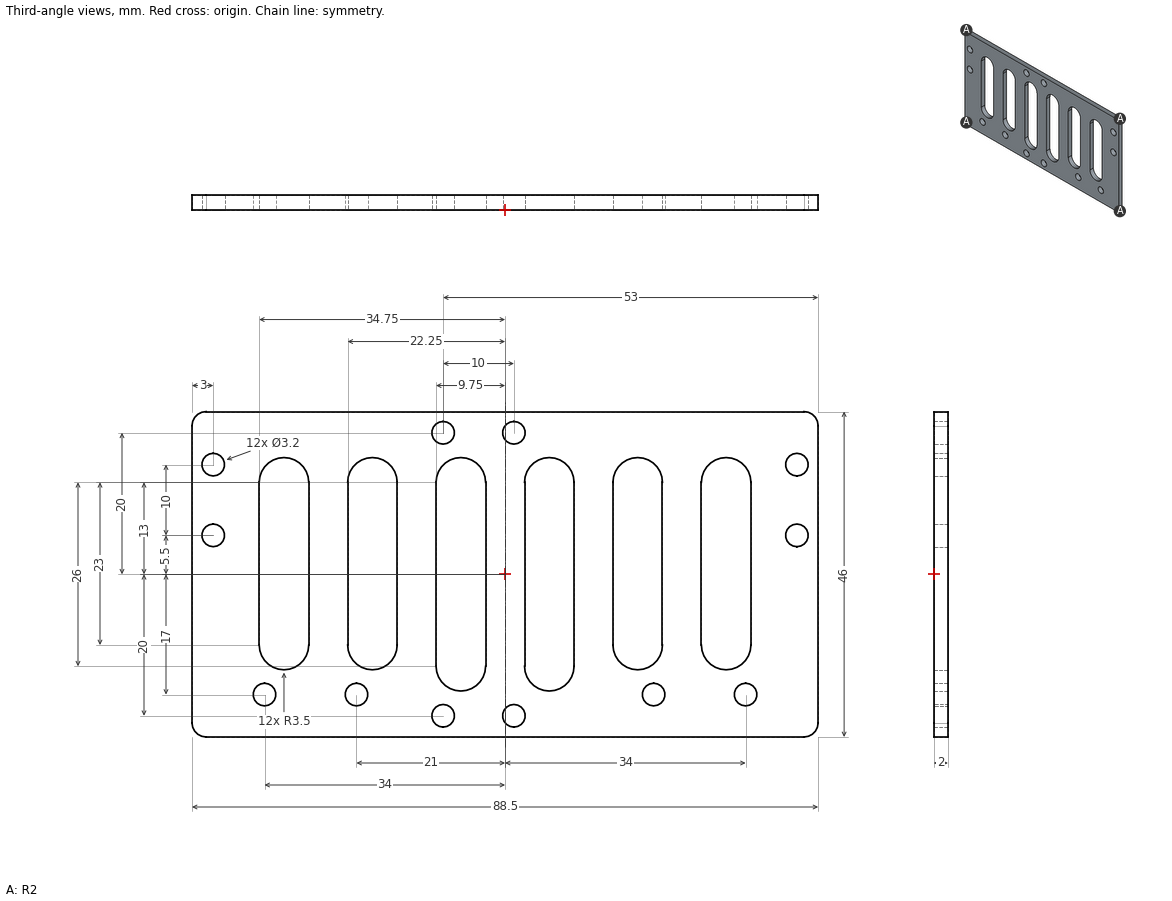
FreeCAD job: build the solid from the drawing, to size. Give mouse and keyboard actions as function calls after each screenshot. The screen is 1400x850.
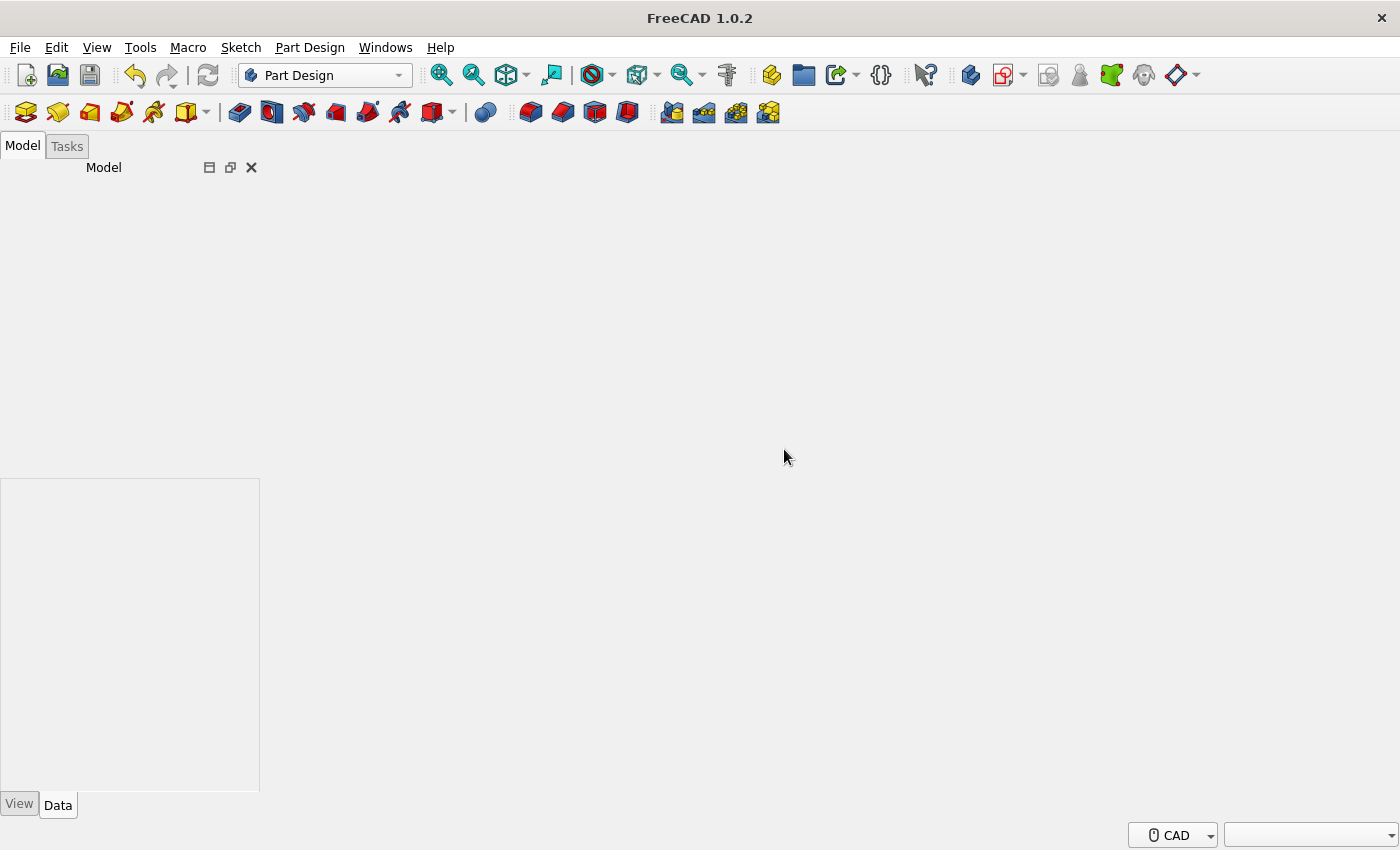
click(26, 76)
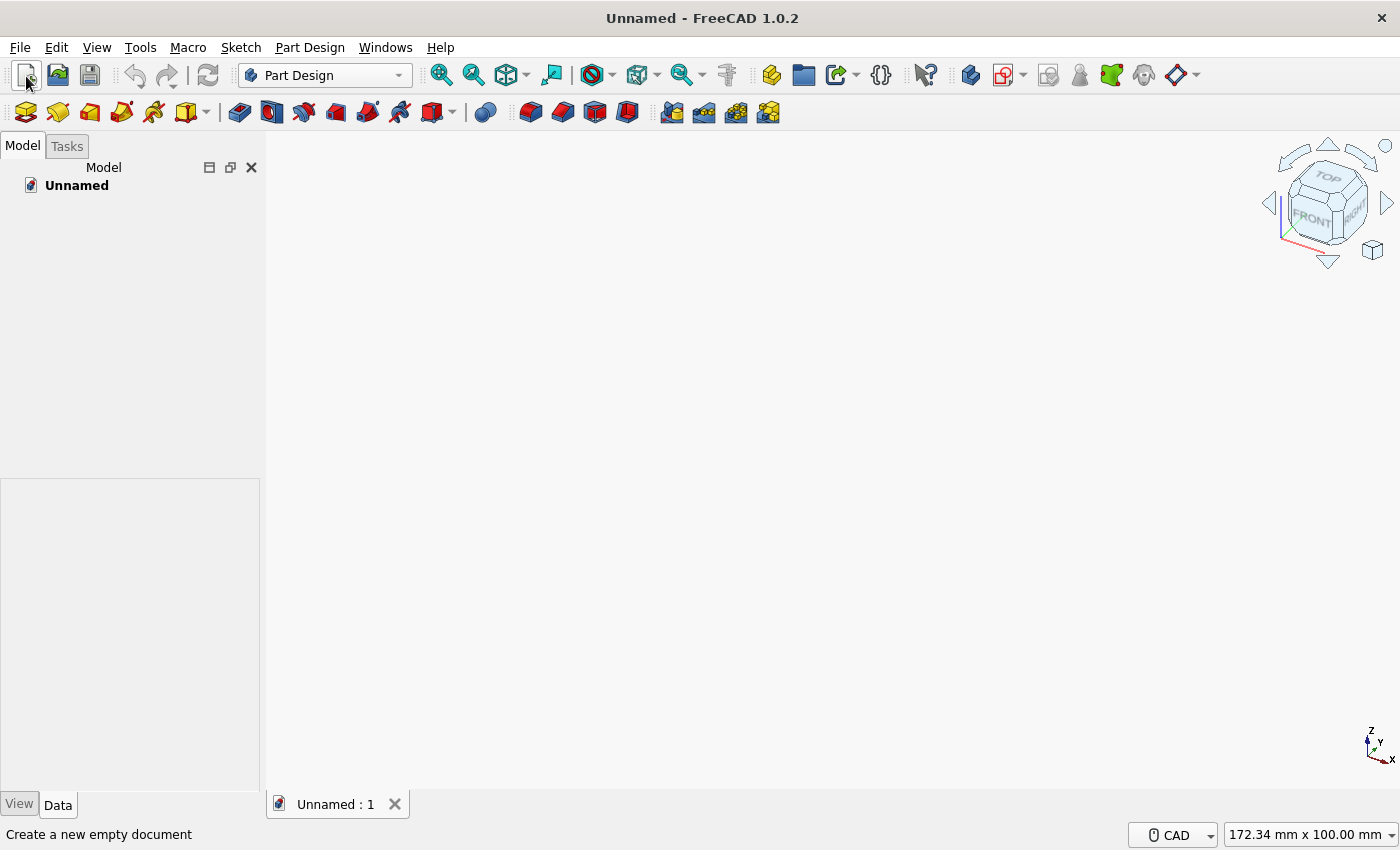
click(1004, 76)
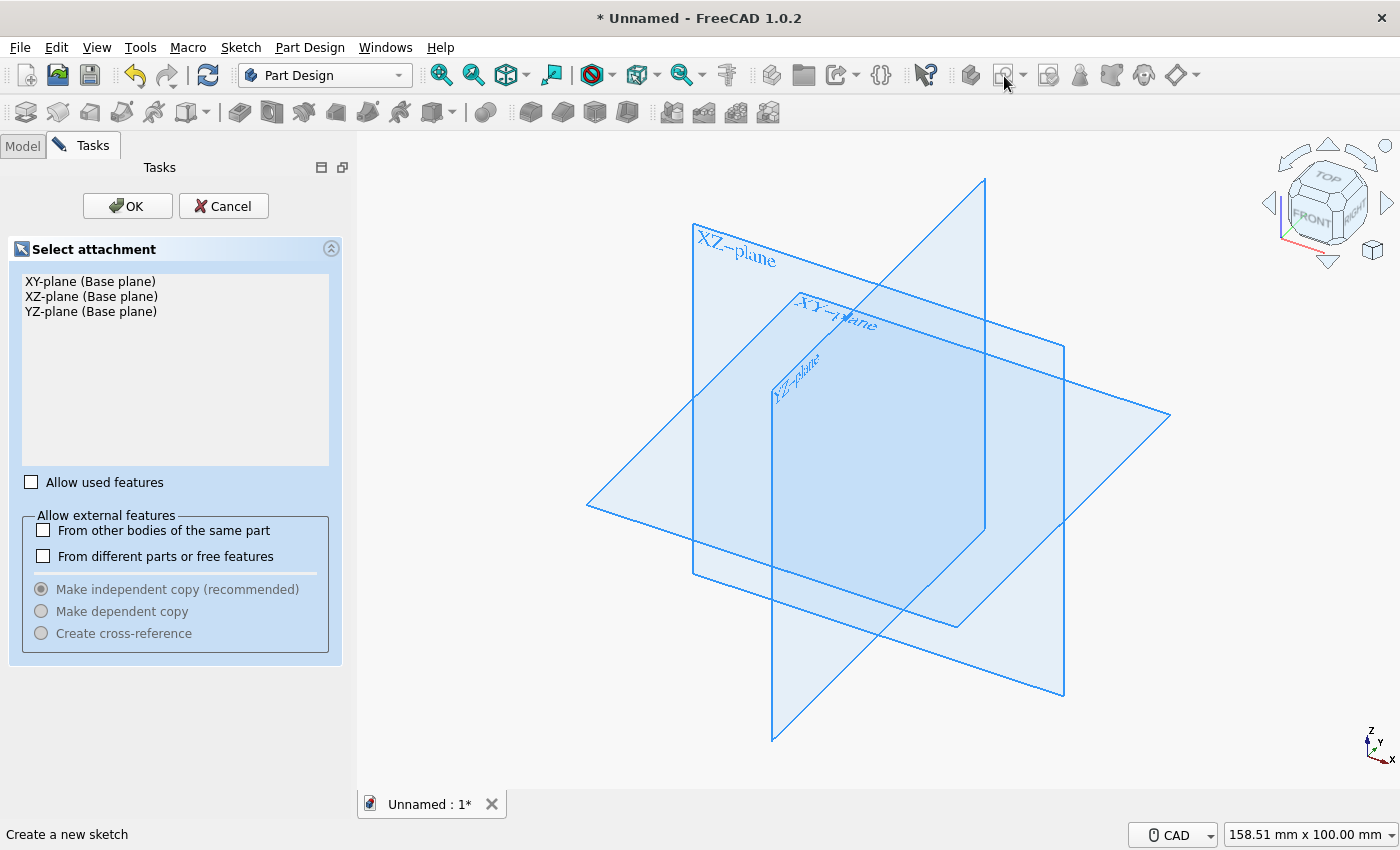
click(82, 296)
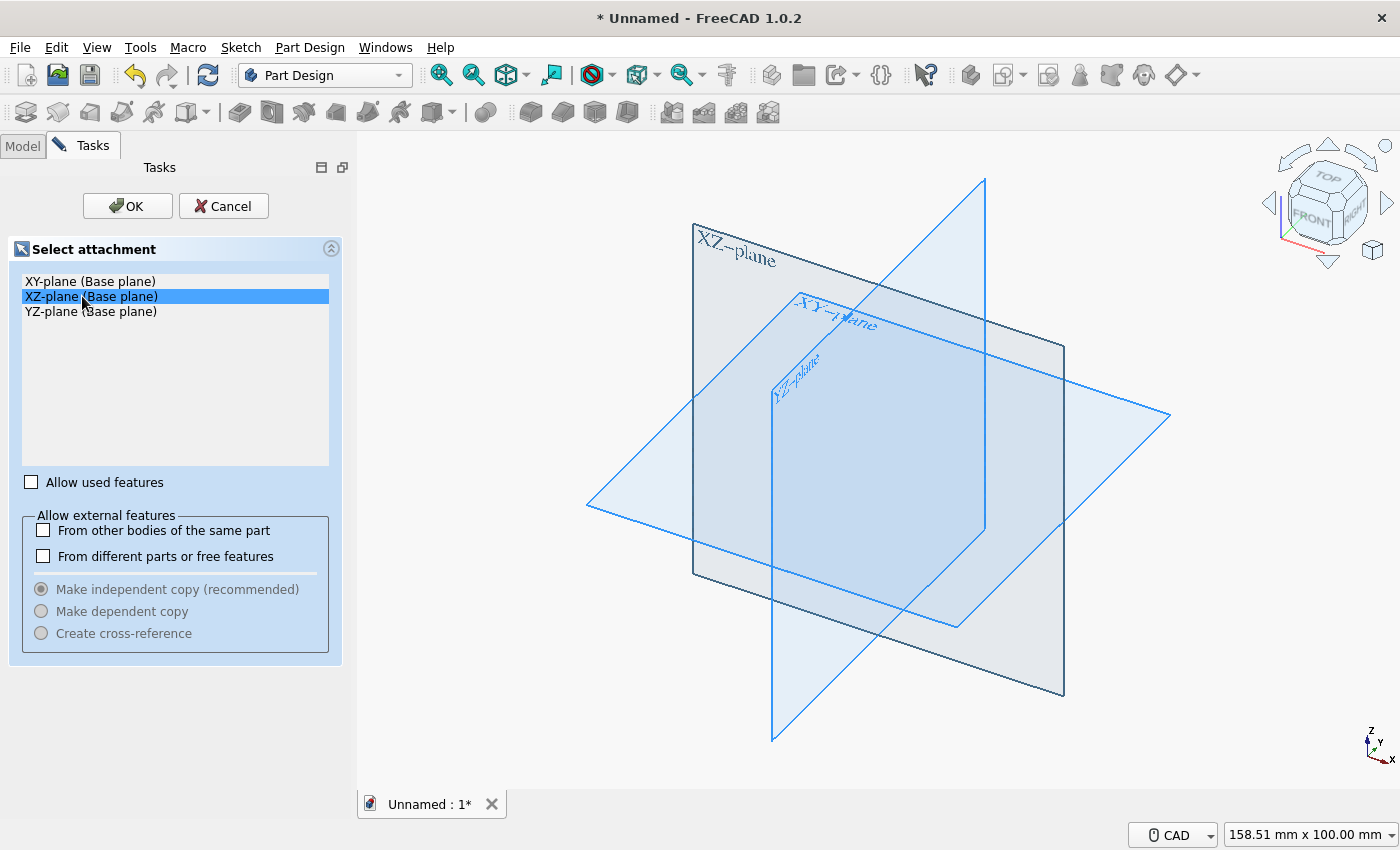
click(128, 206)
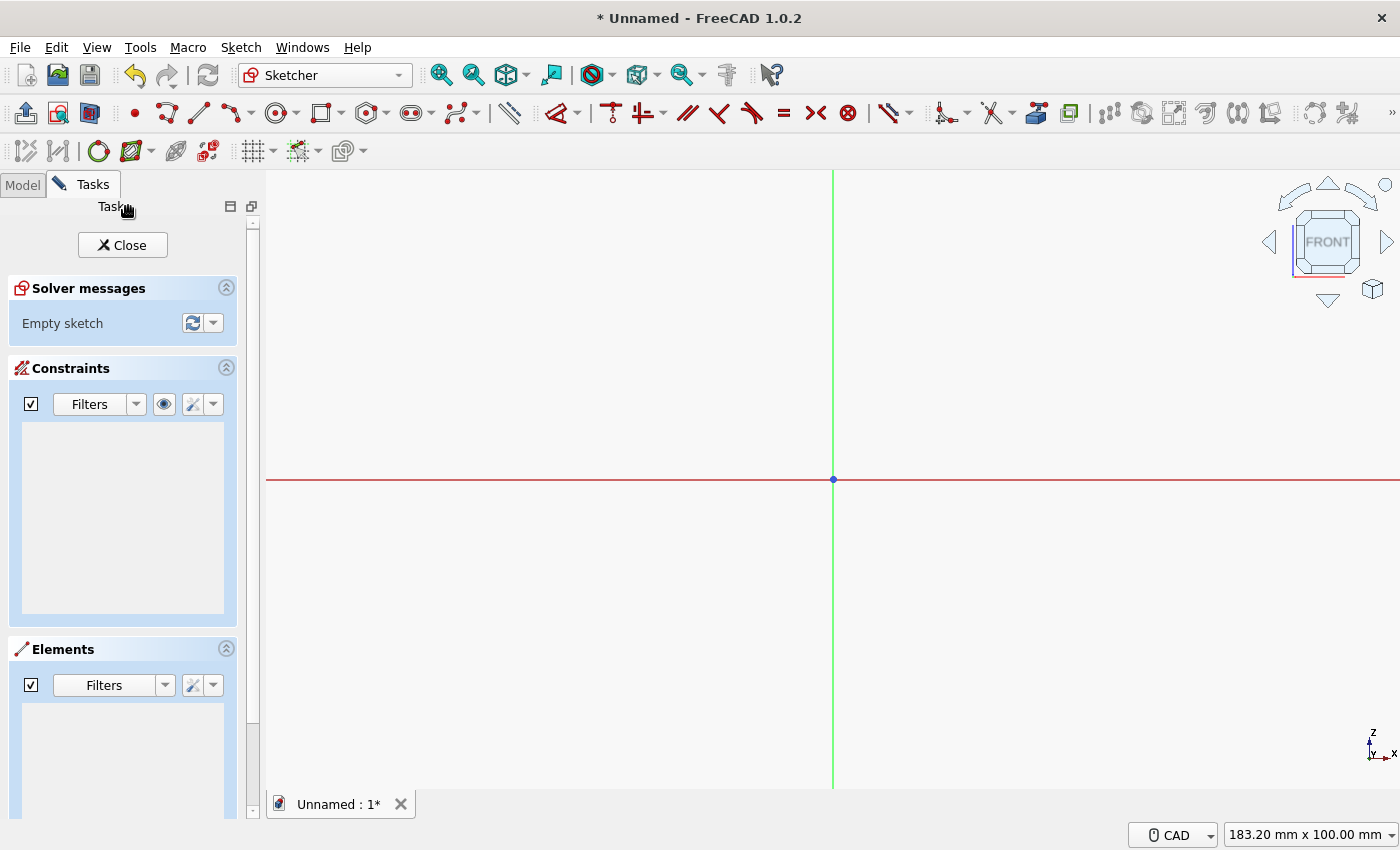
key(g)
key(v)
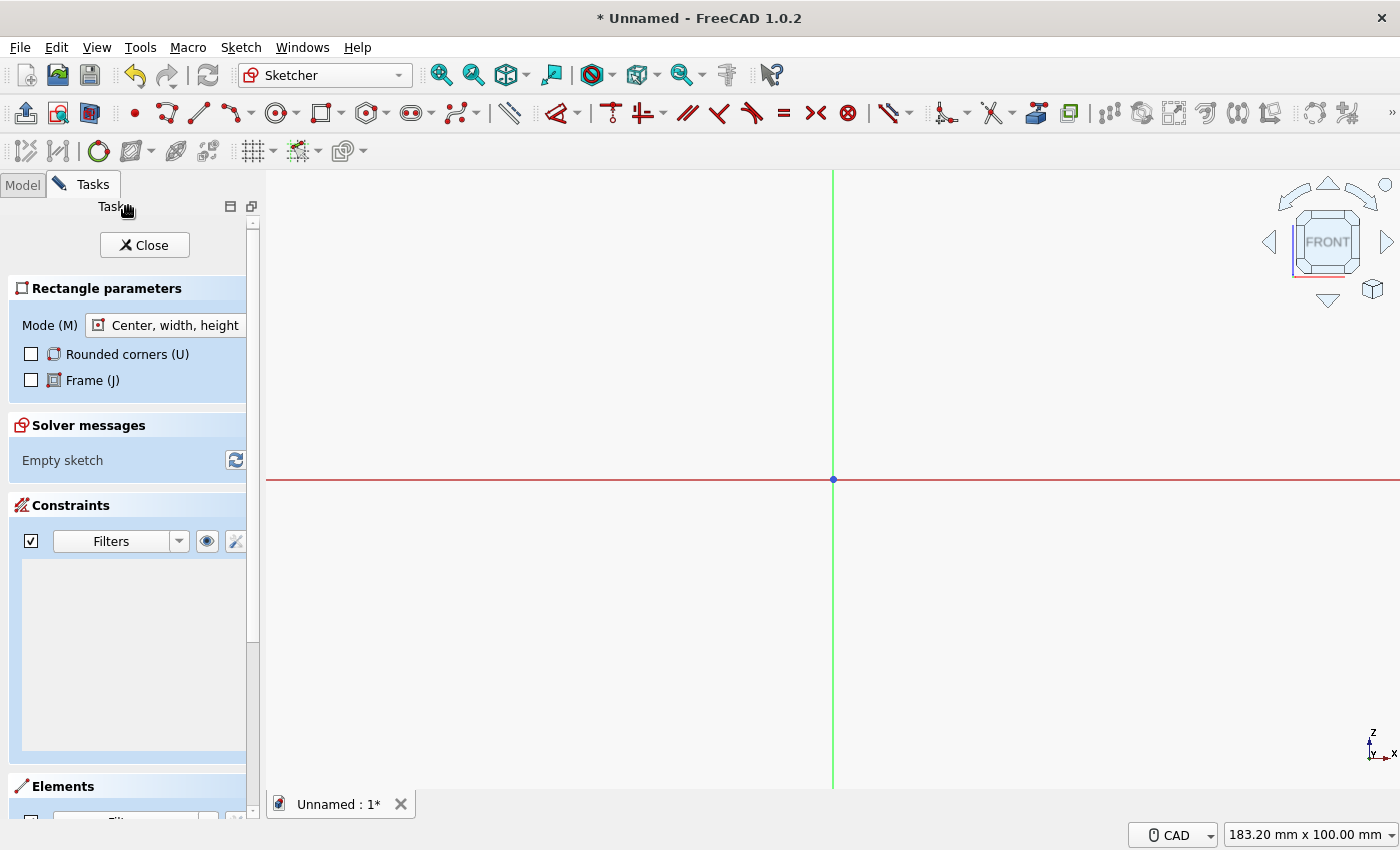
click(833, 480)
click(1107, 337)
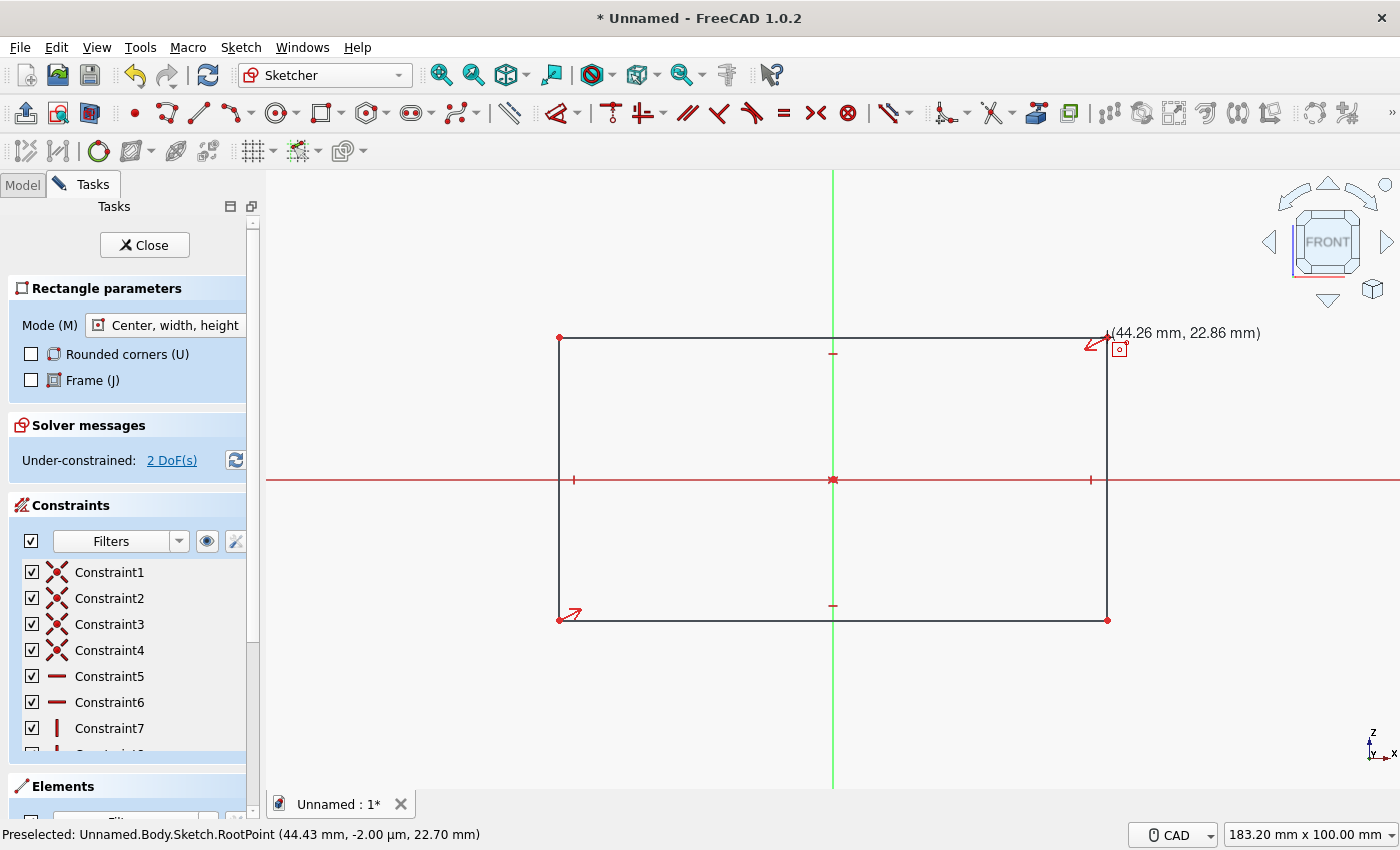
click(276, 114)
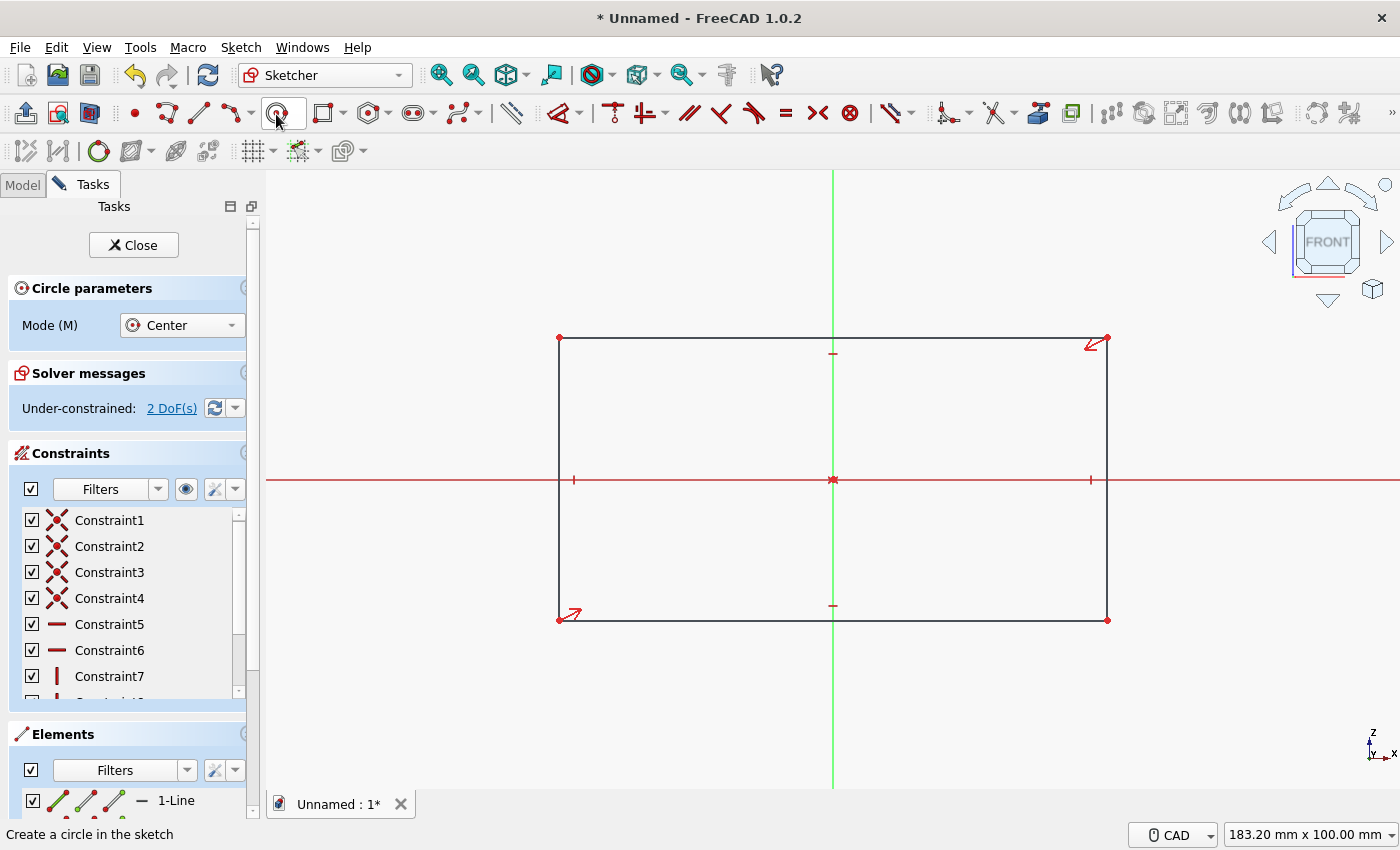
scroll(578, 384, up, 5)